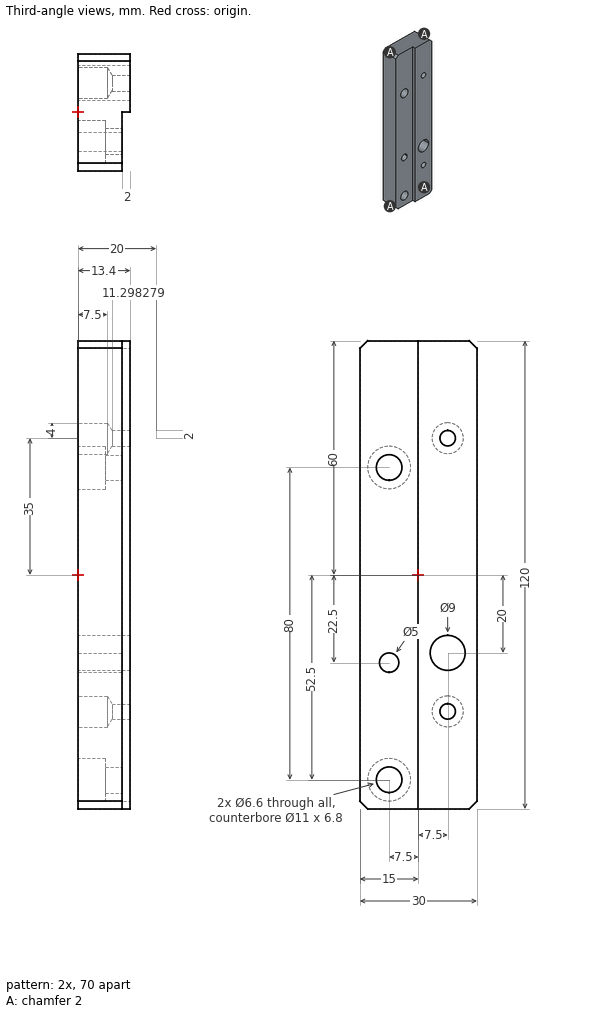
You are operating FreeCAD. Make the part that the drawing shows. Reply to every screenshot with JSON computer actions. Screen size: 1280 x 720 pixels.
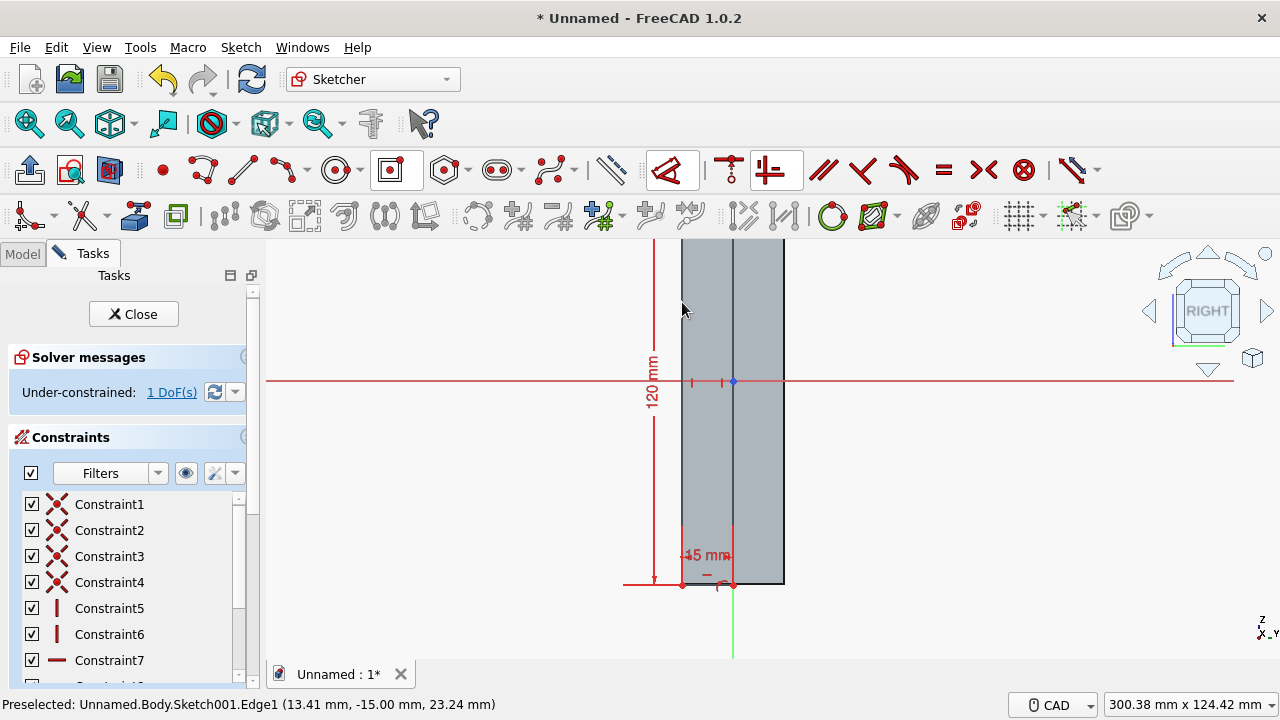
{"action": "scroll", "coordinate": [698, 586], "scroll_direction": "down", "scroll_amount": 2}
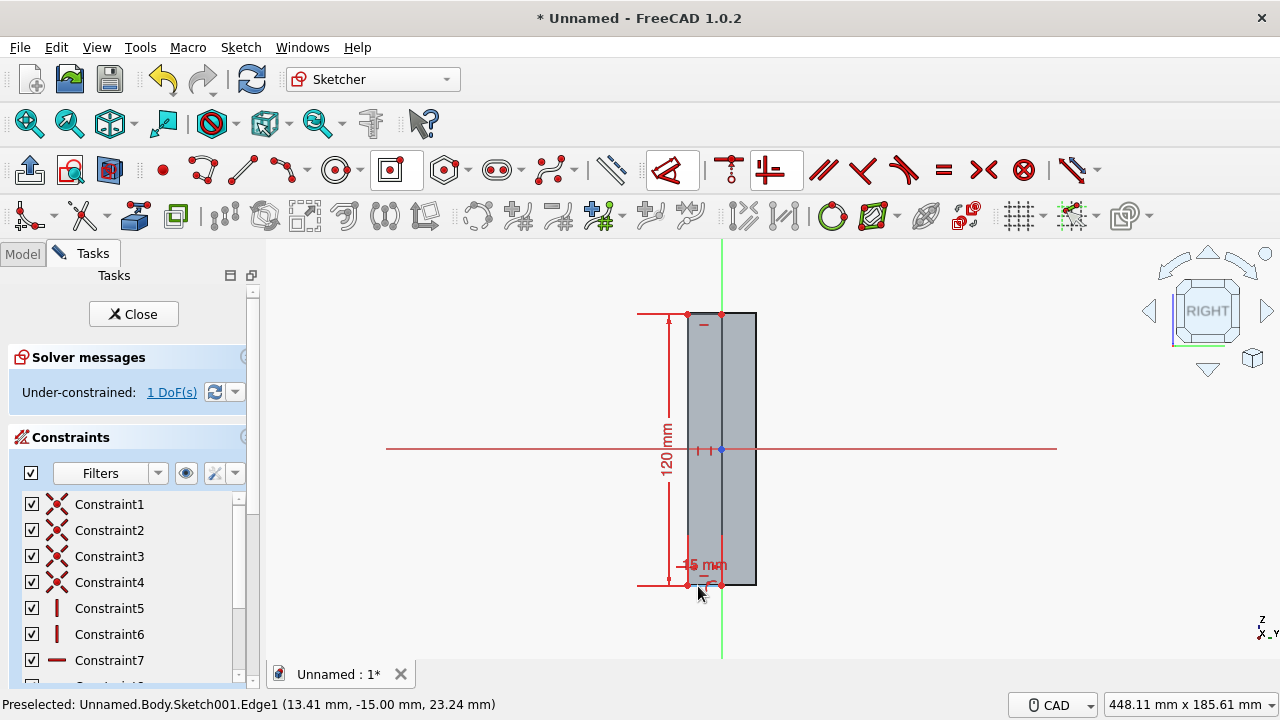
{"action": "left_click", "coordinate": [688, 314]}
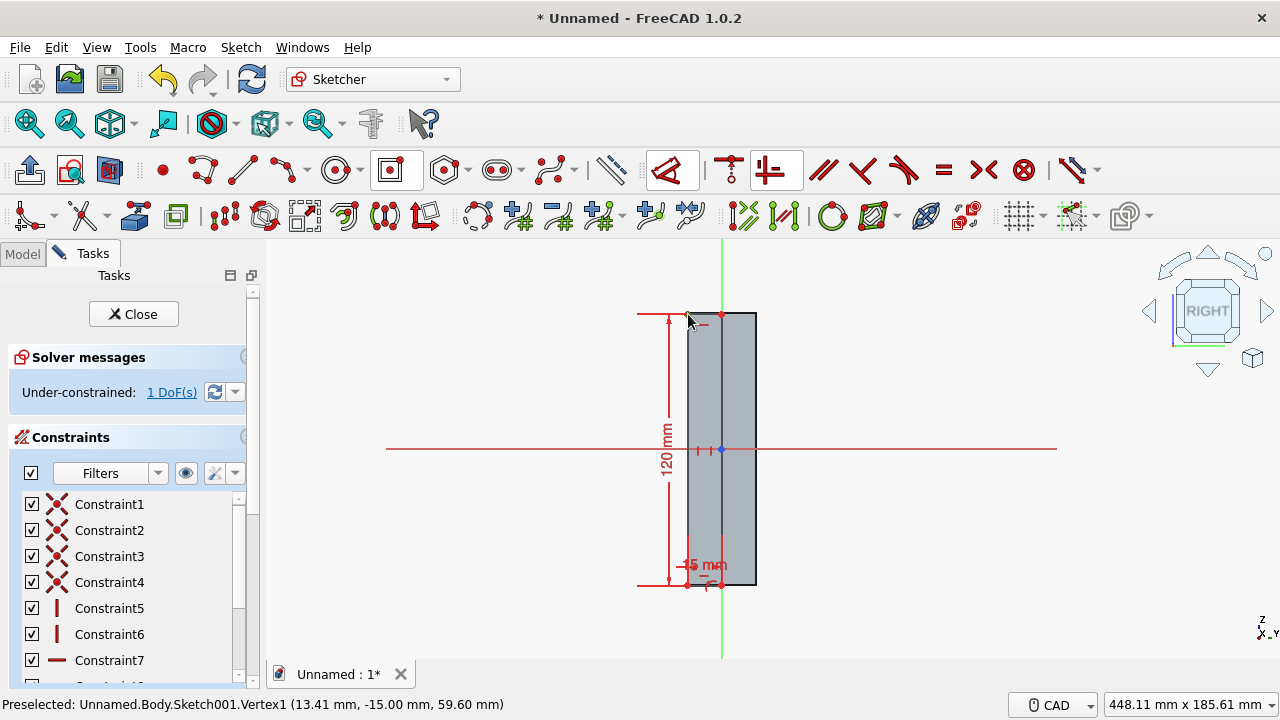
{"action": "left_click", "coordinate": [694, 170]}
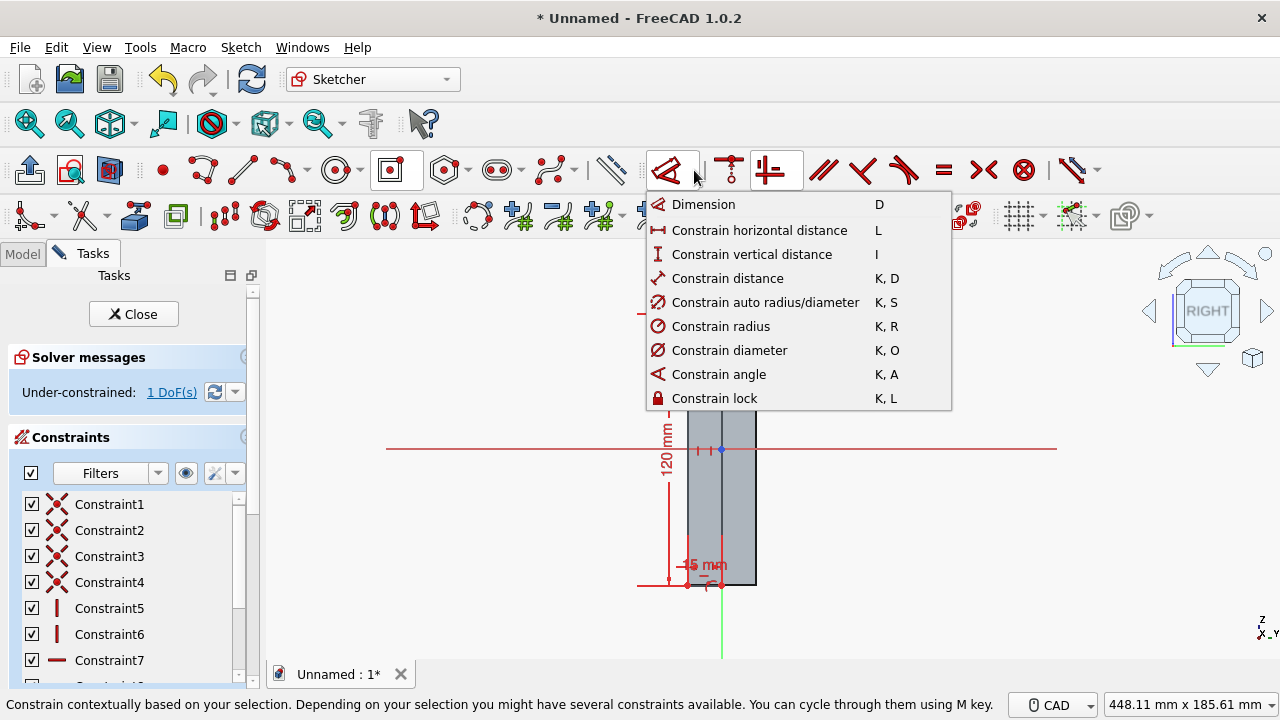
{"action": "left_click", "coordinate": [799, 254]}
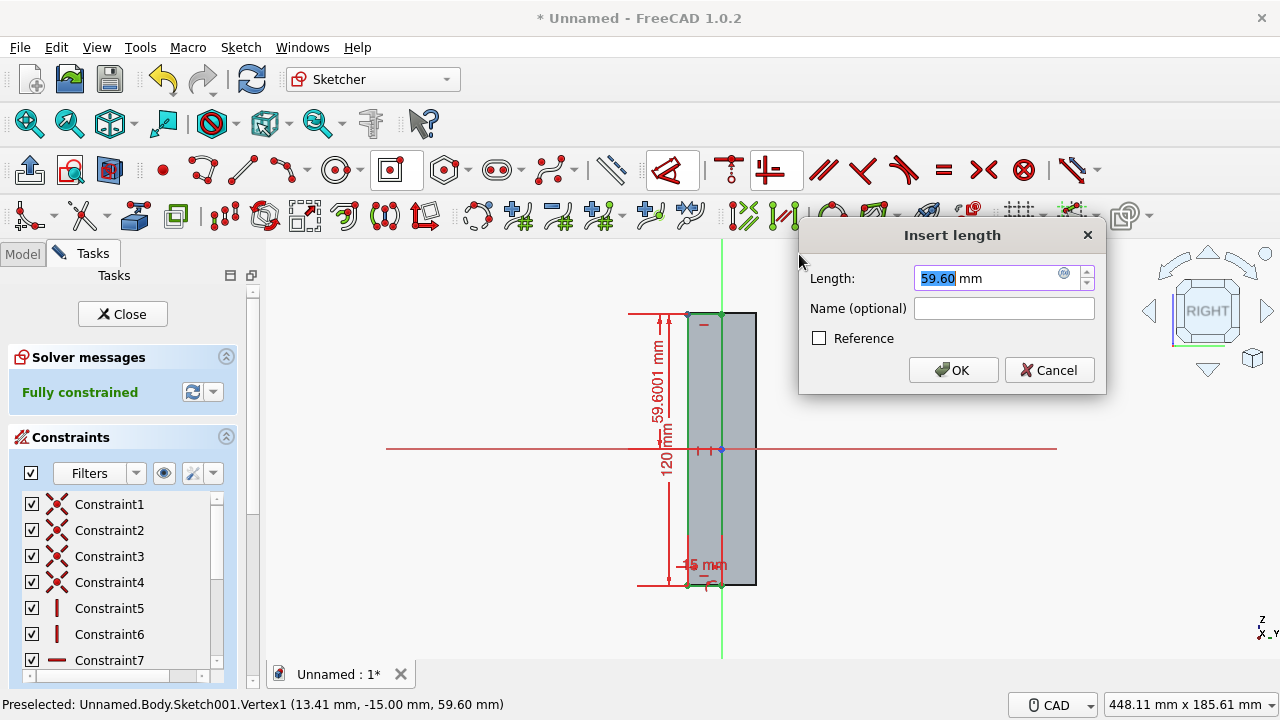
{"action": "type", "text": "60"}
{"action": "key", "text": "Return"}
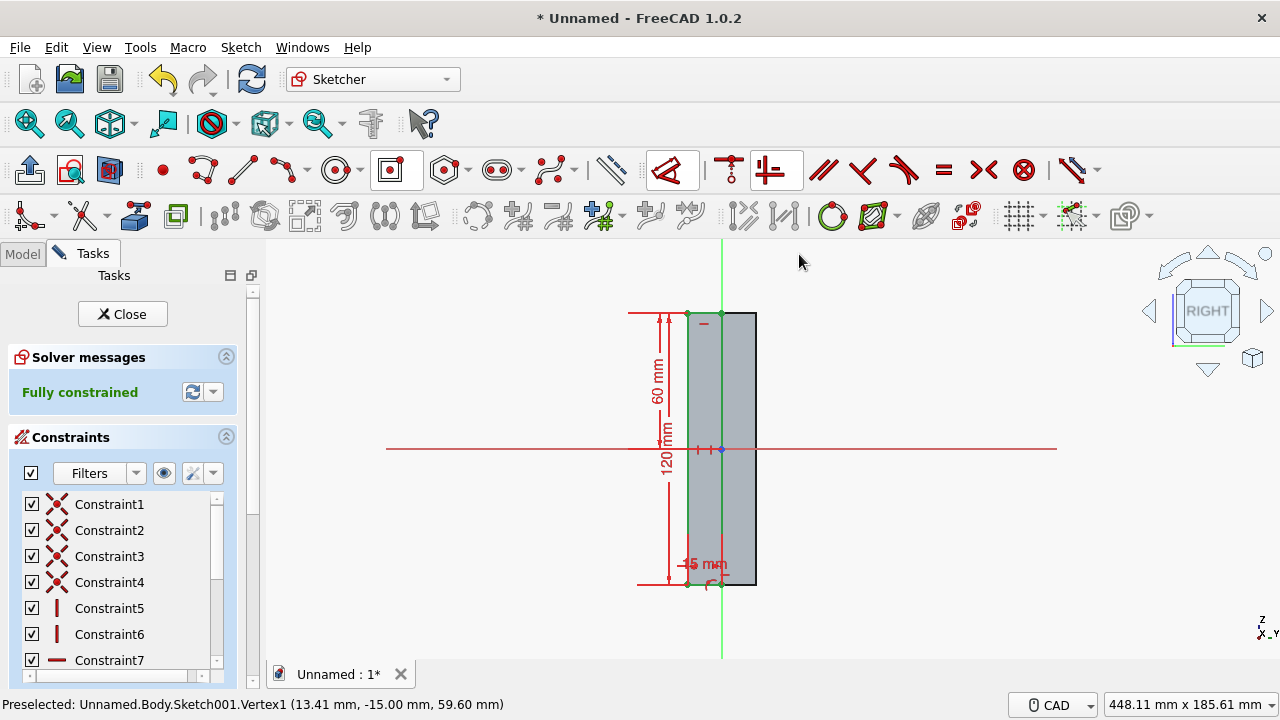
{"action": "left_click", "coordinate": [123, 314]}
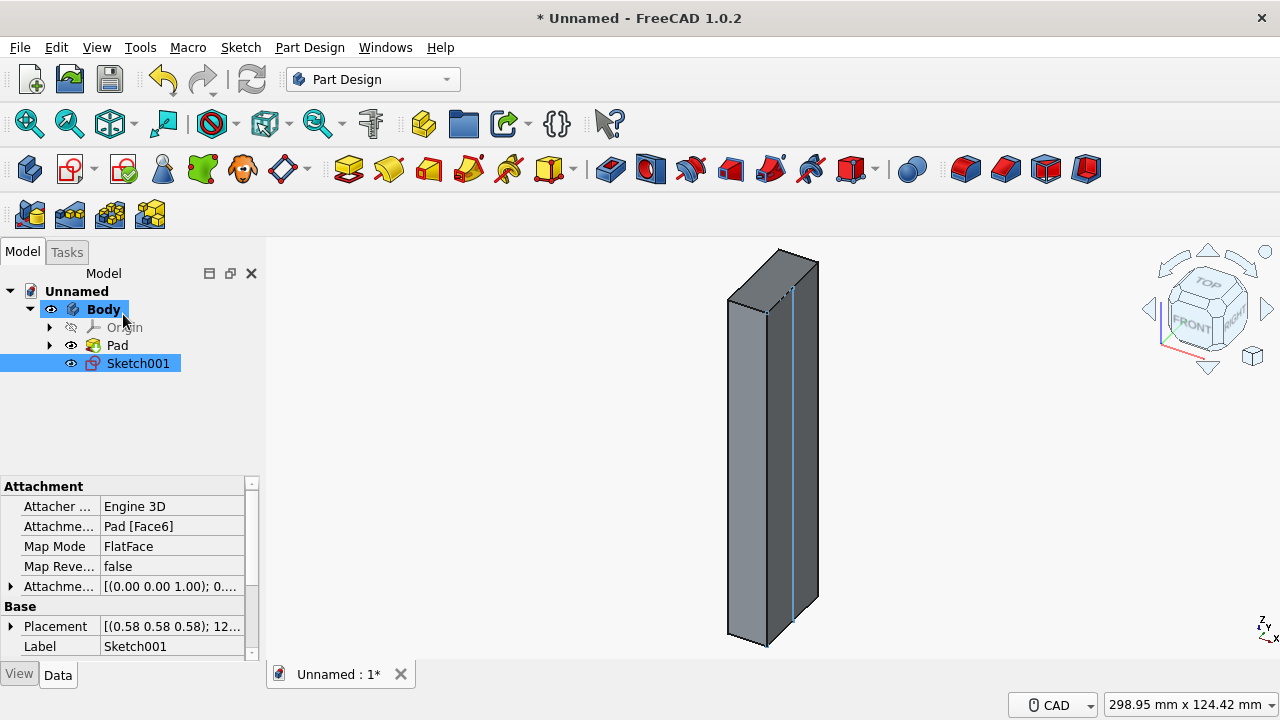
{"action": "left_click", "coordinate": [612, 170]}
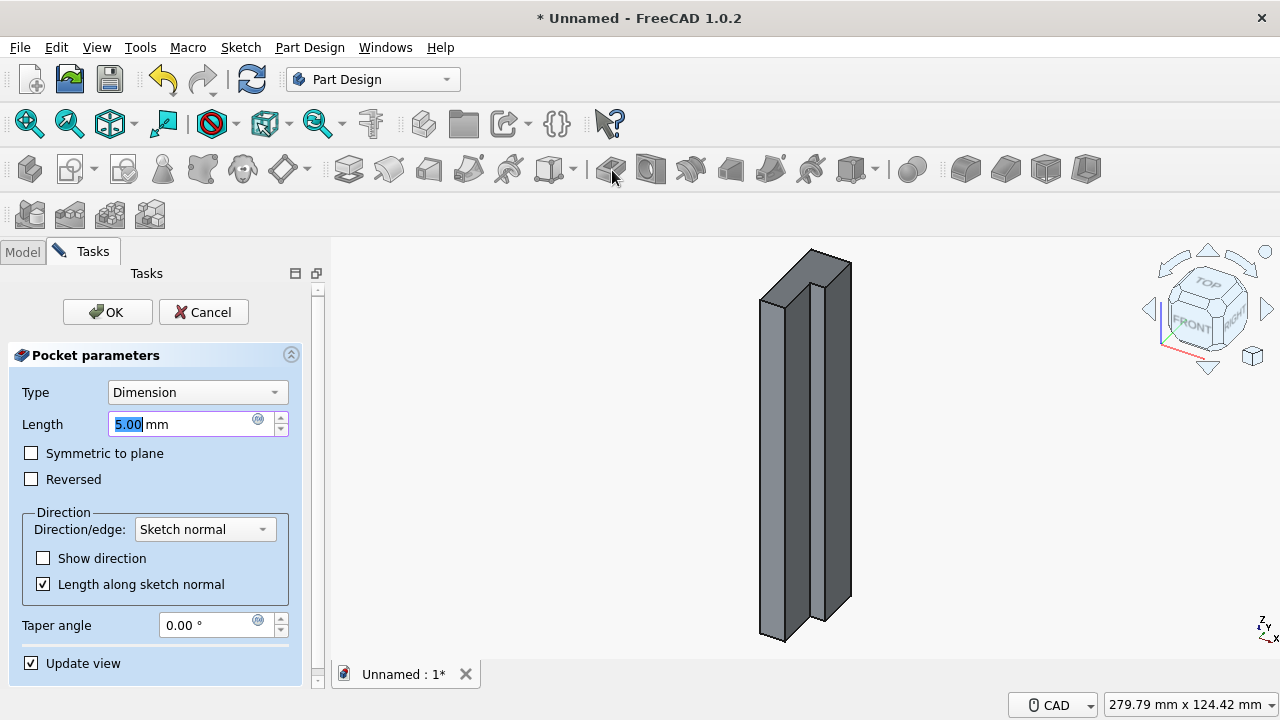
{"action": "type", "text": "2"}
{"action": "key", "text": "Tab"}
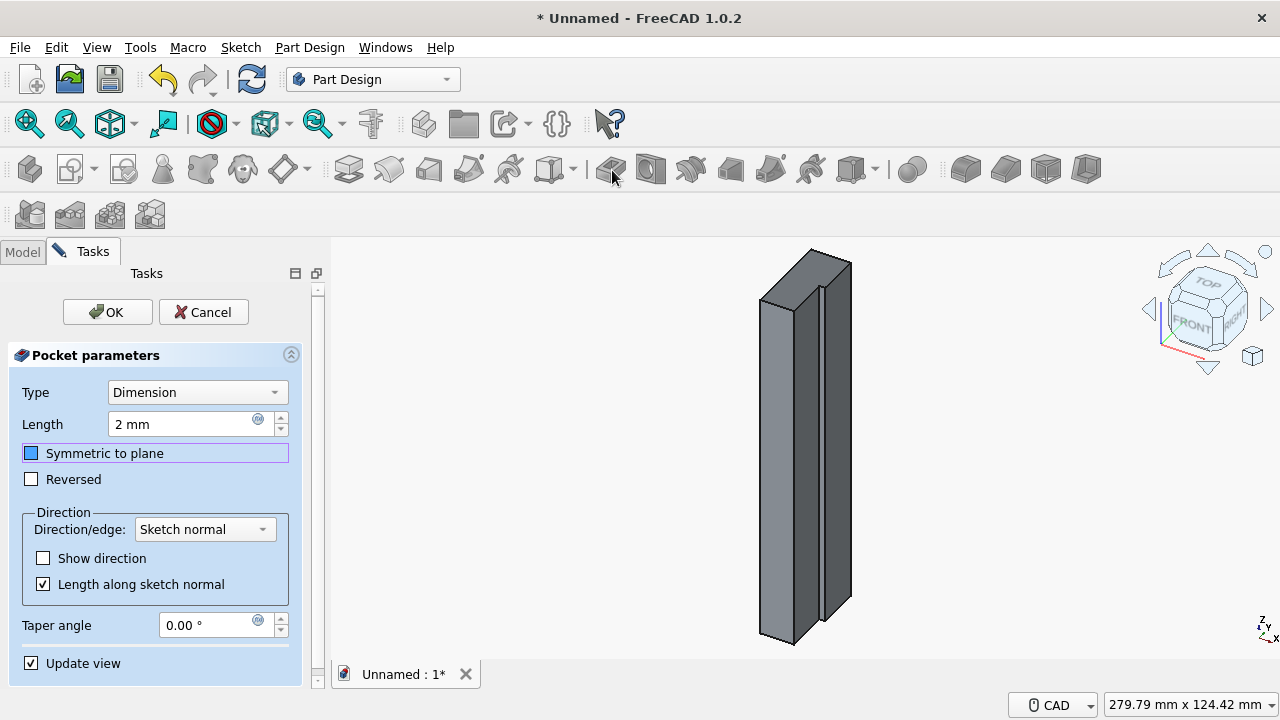
{"action": "left_click", "coordinate": [108, 312]}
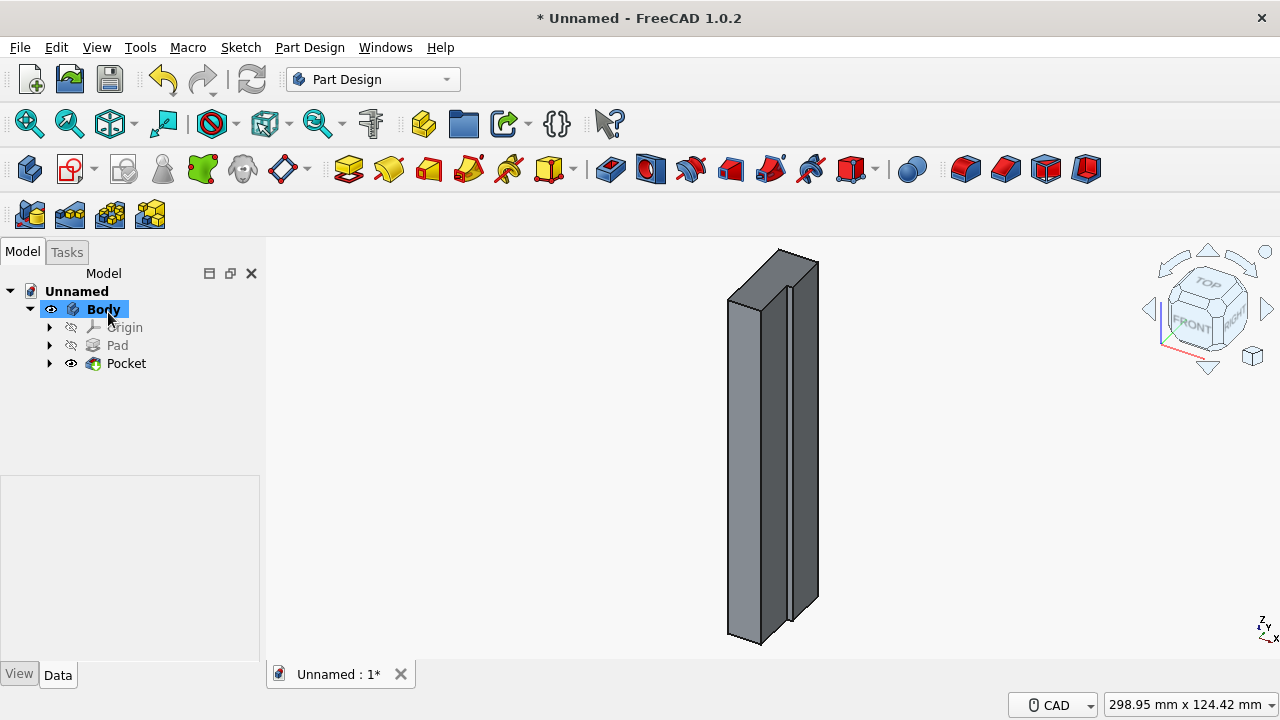
{"action": "left_click", "coordinate": [50, 327]}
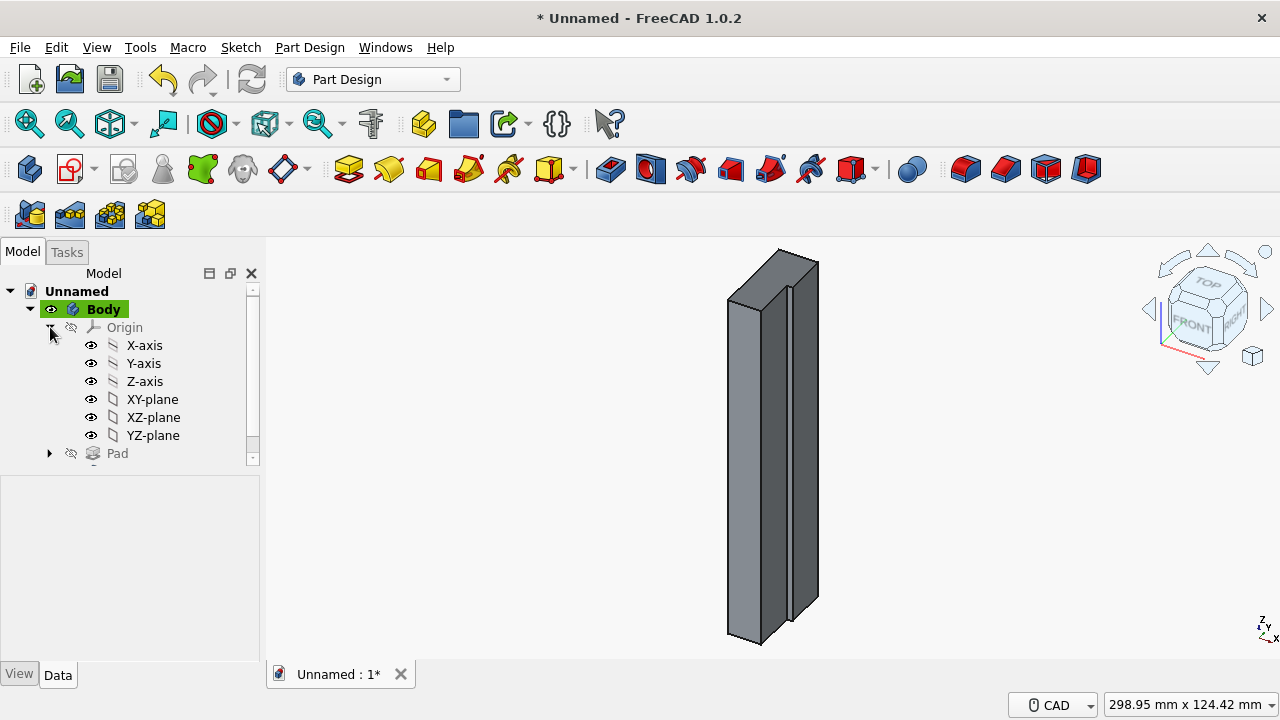
{"action": "left_click", "coordinate": [136, 417]}